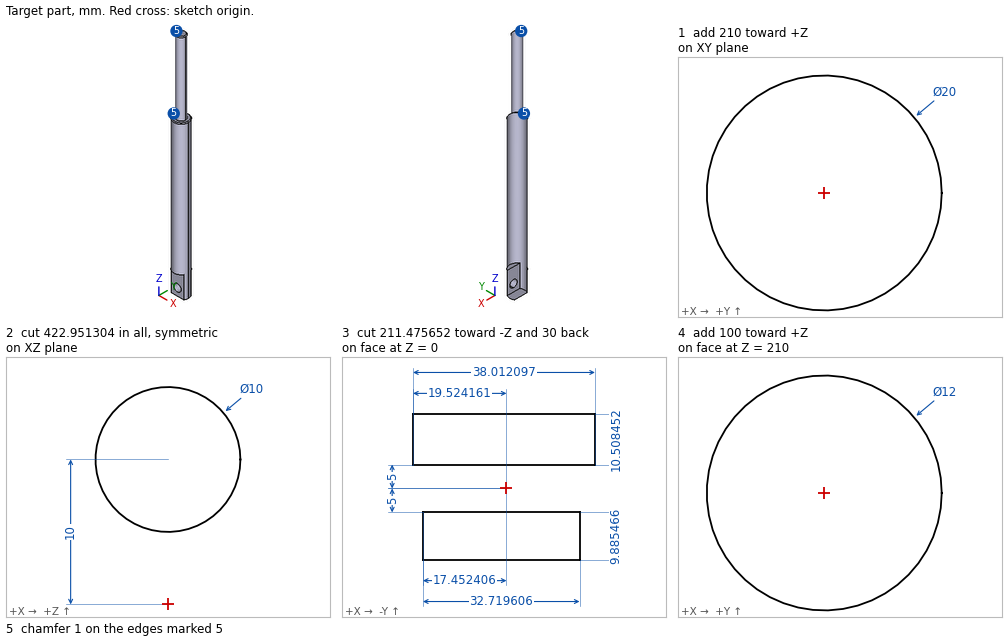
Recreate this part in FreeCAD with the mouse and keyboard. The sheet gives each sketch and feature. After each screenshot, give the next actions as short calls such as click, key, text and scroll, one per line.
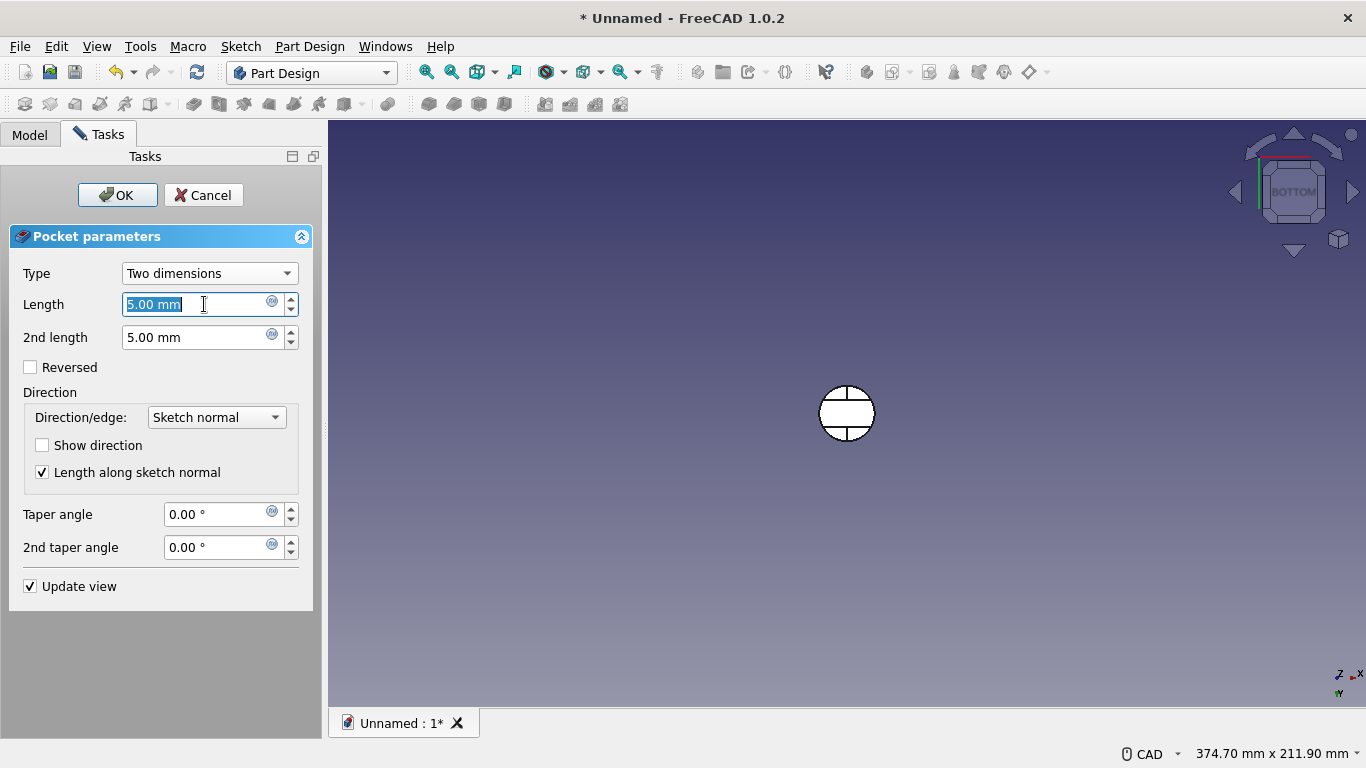
text(211.475652)
key(Tab)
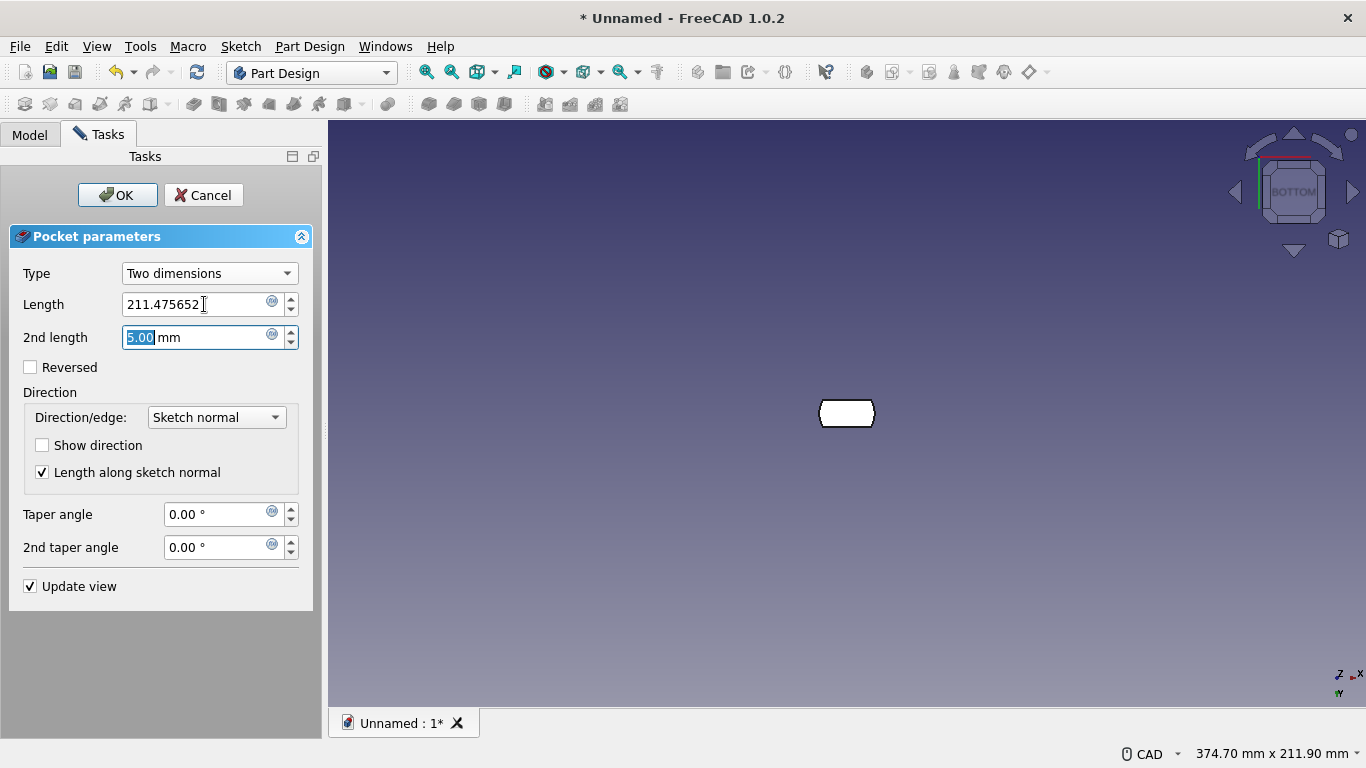
text(30)
key(Tab)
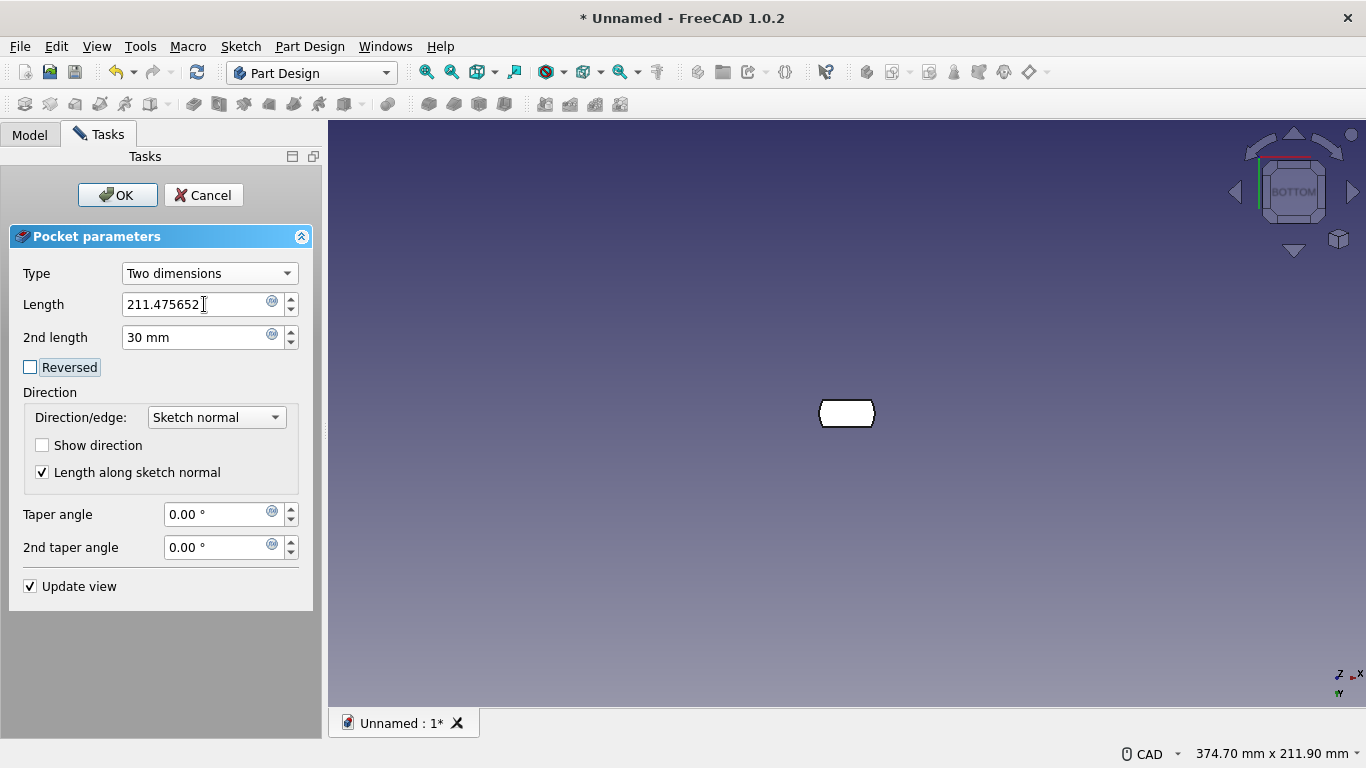
click(31, 367)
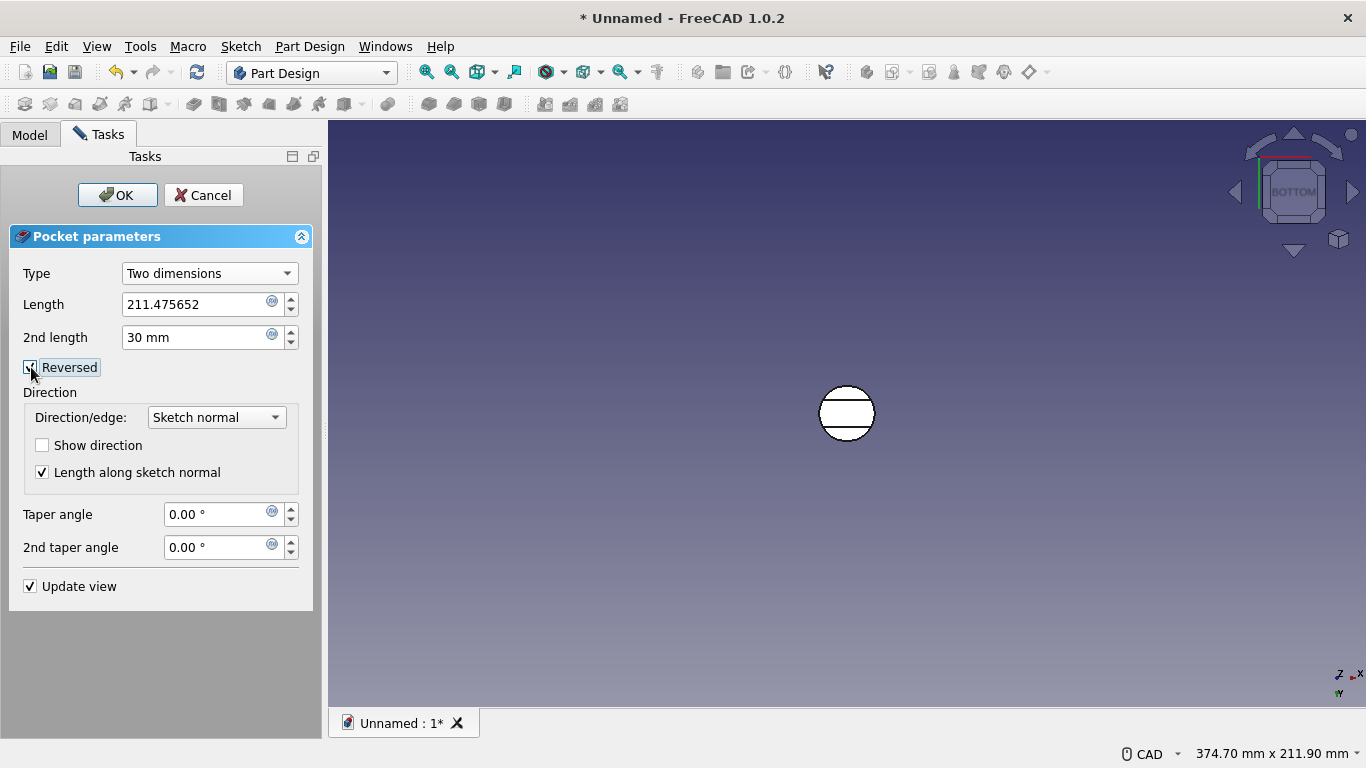
click(118, 195)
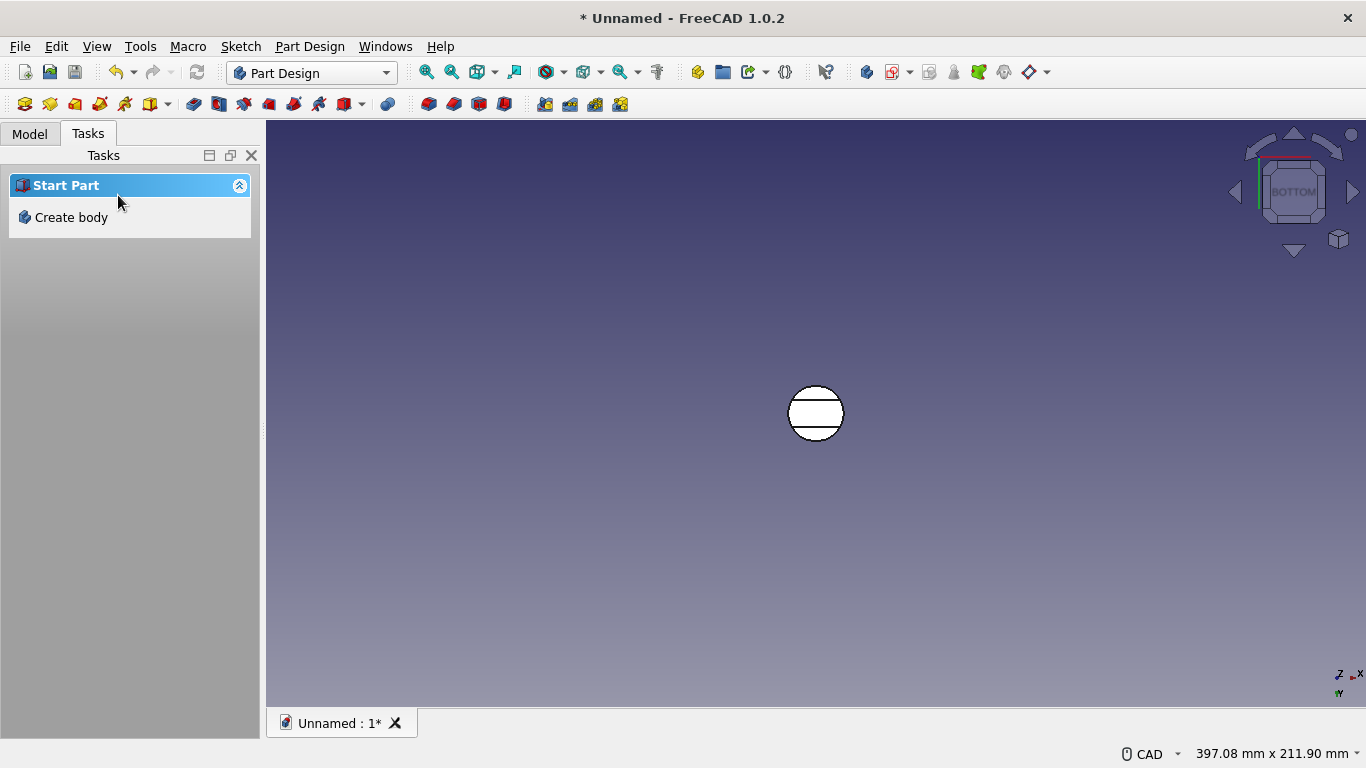
click(427, 72)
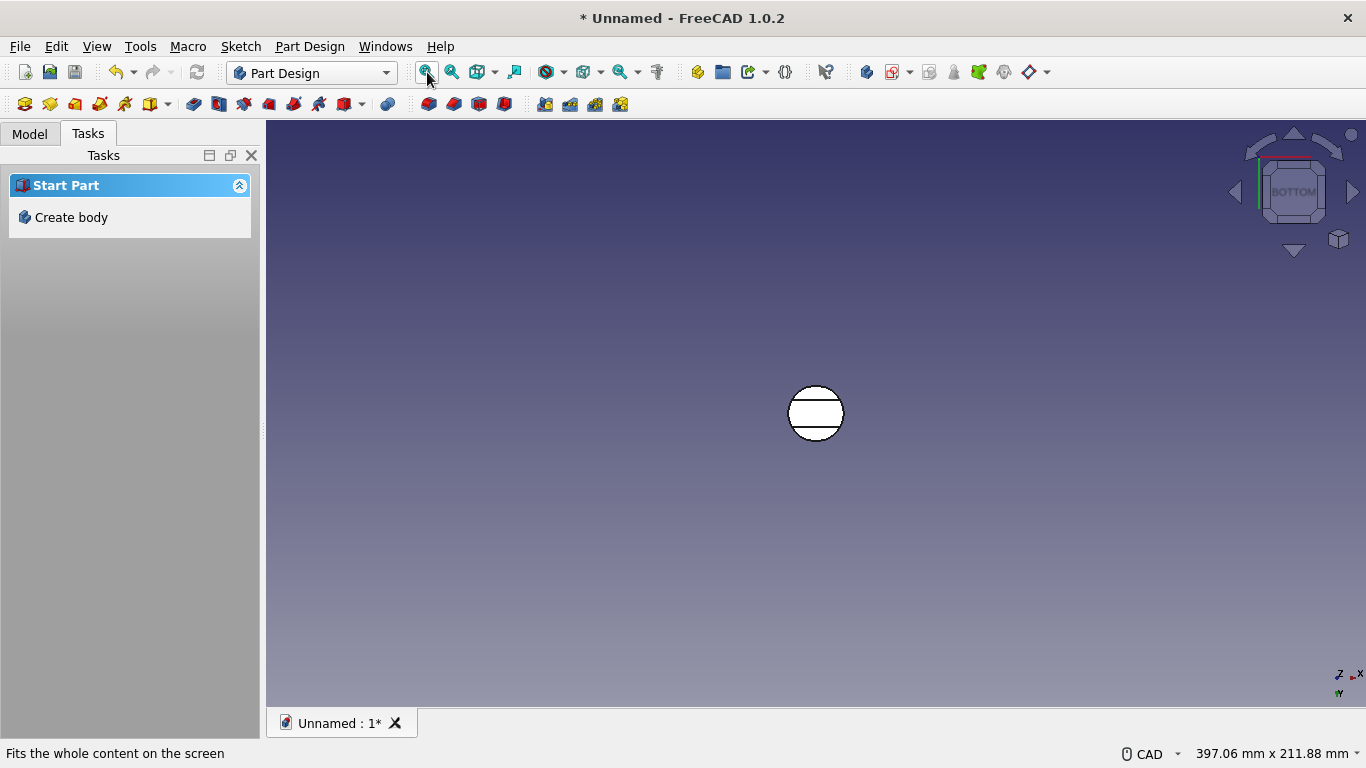
key(0)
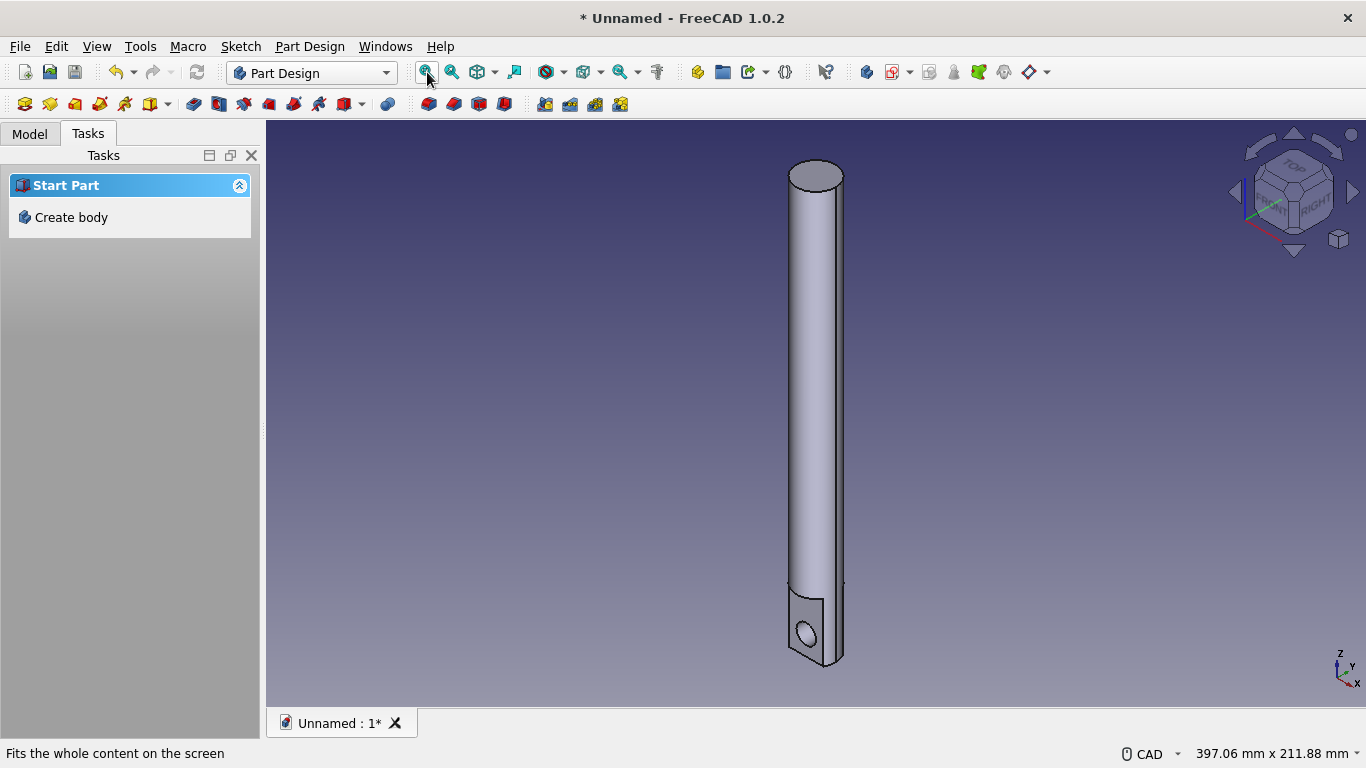
click(816, 175)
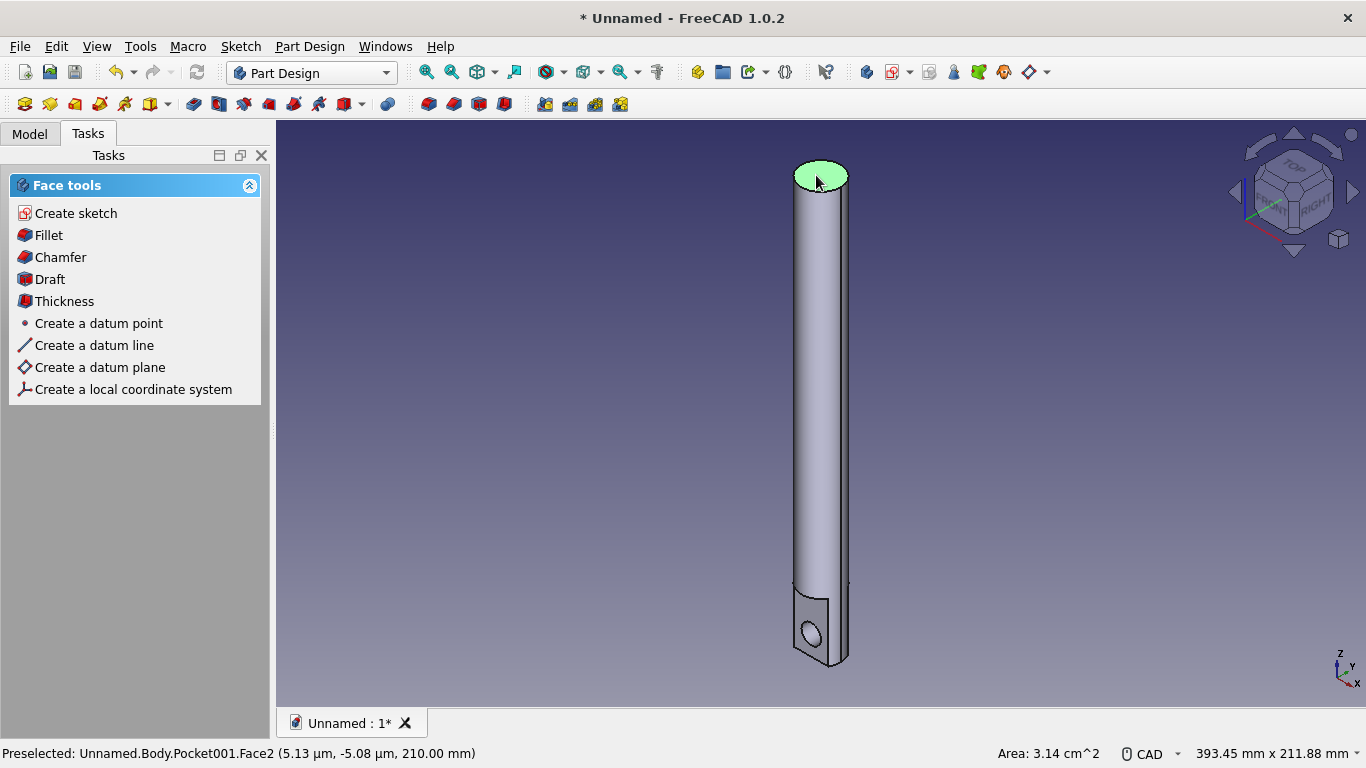
click(892, 72)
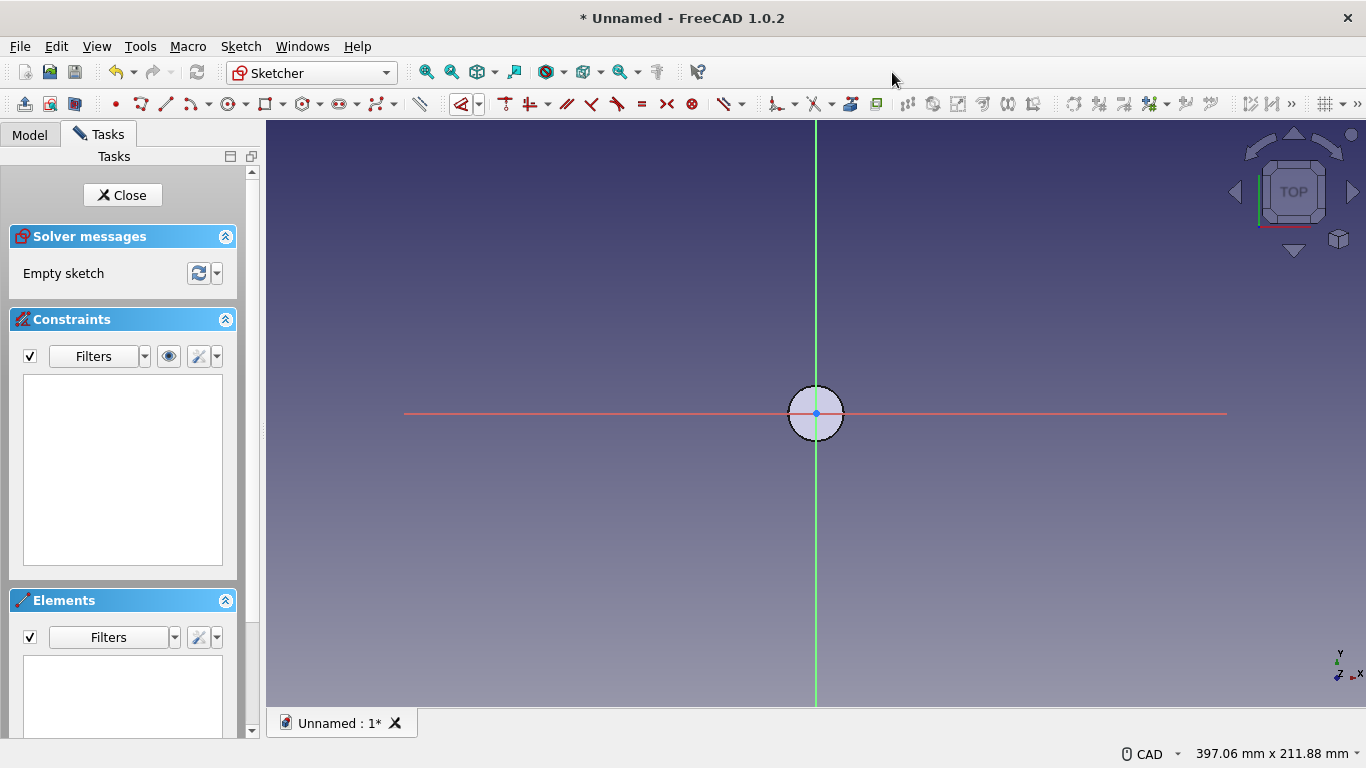
scroll(823, 414, up, 12)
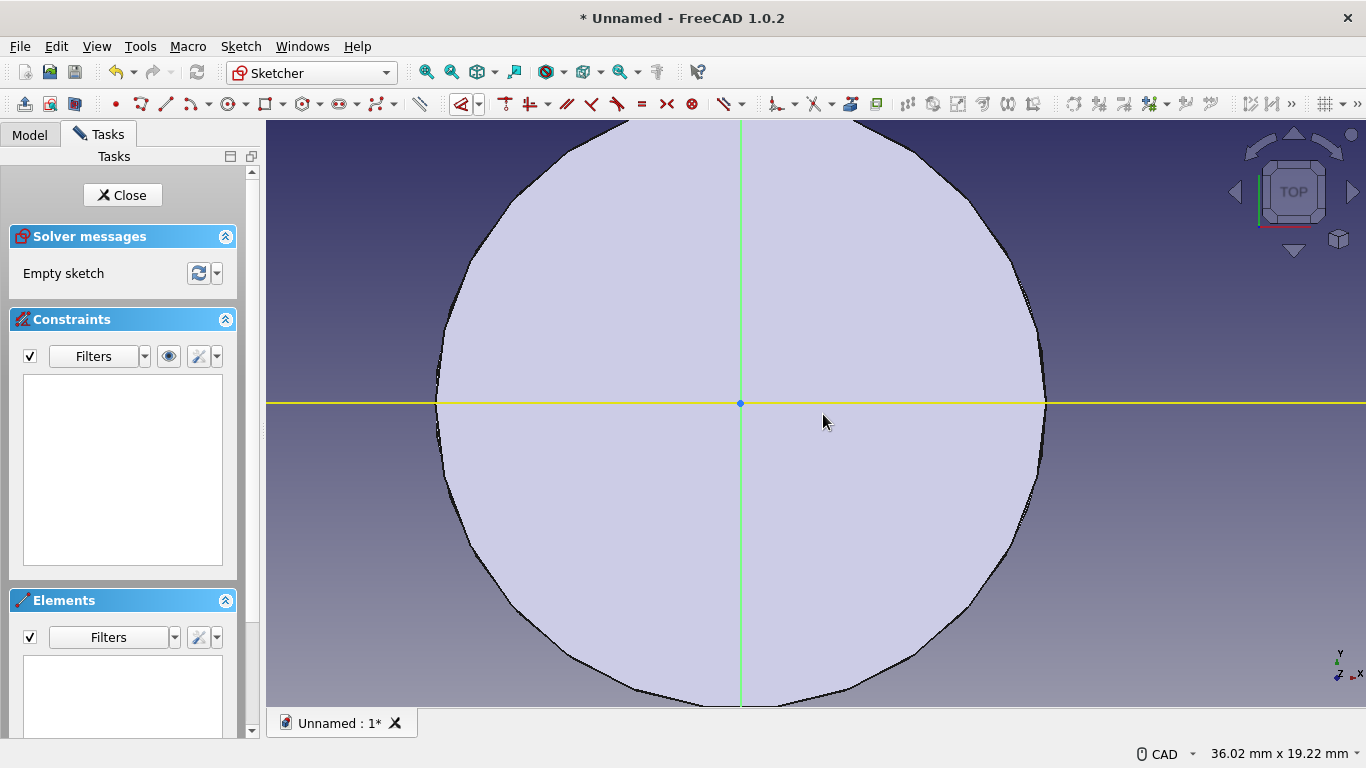
click(228, 104)